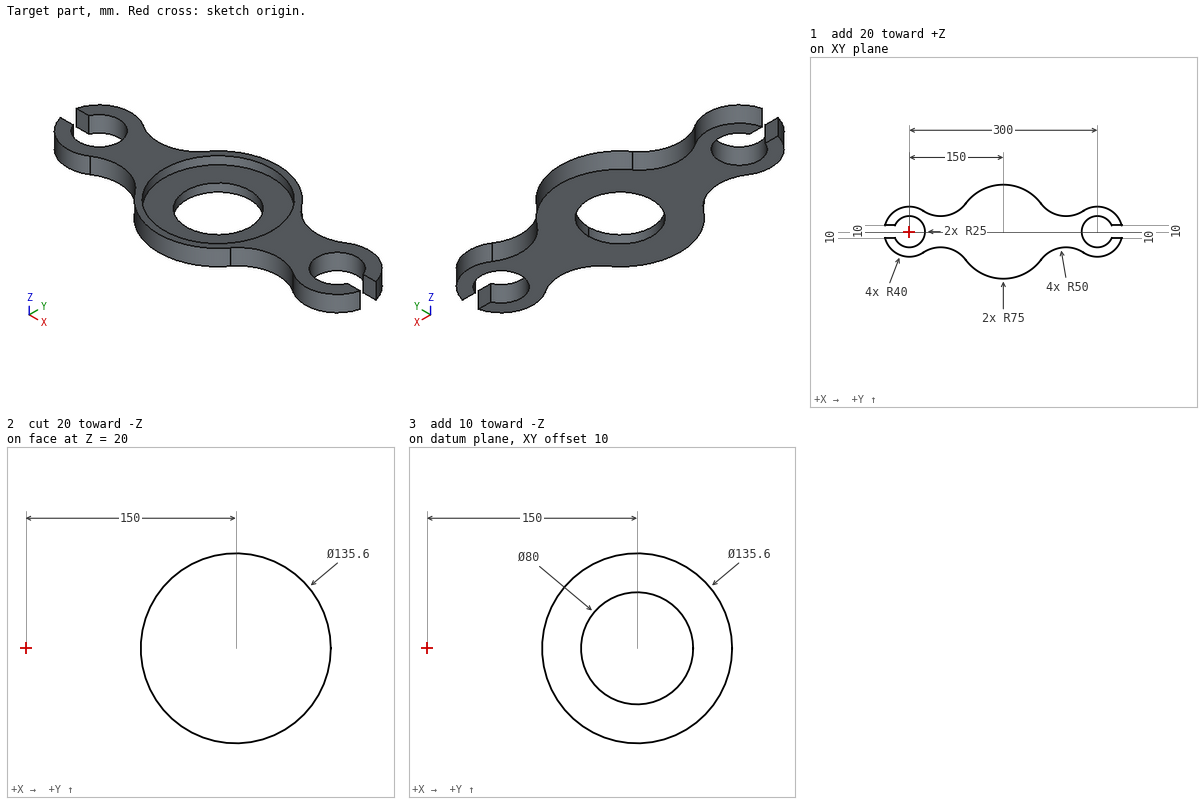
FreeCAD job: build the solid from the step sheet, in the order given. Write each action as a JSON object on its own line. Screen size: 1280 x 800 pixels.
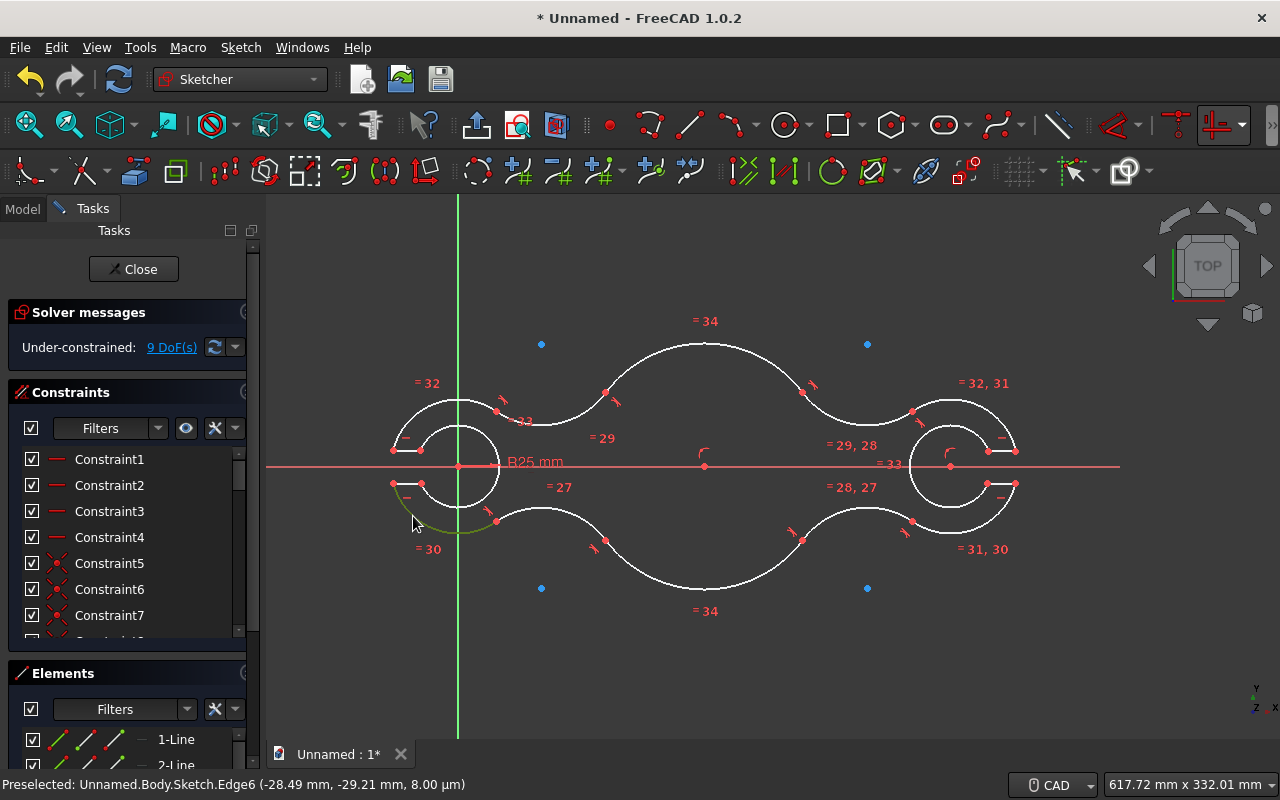
{"action": "key", "text": "k r"}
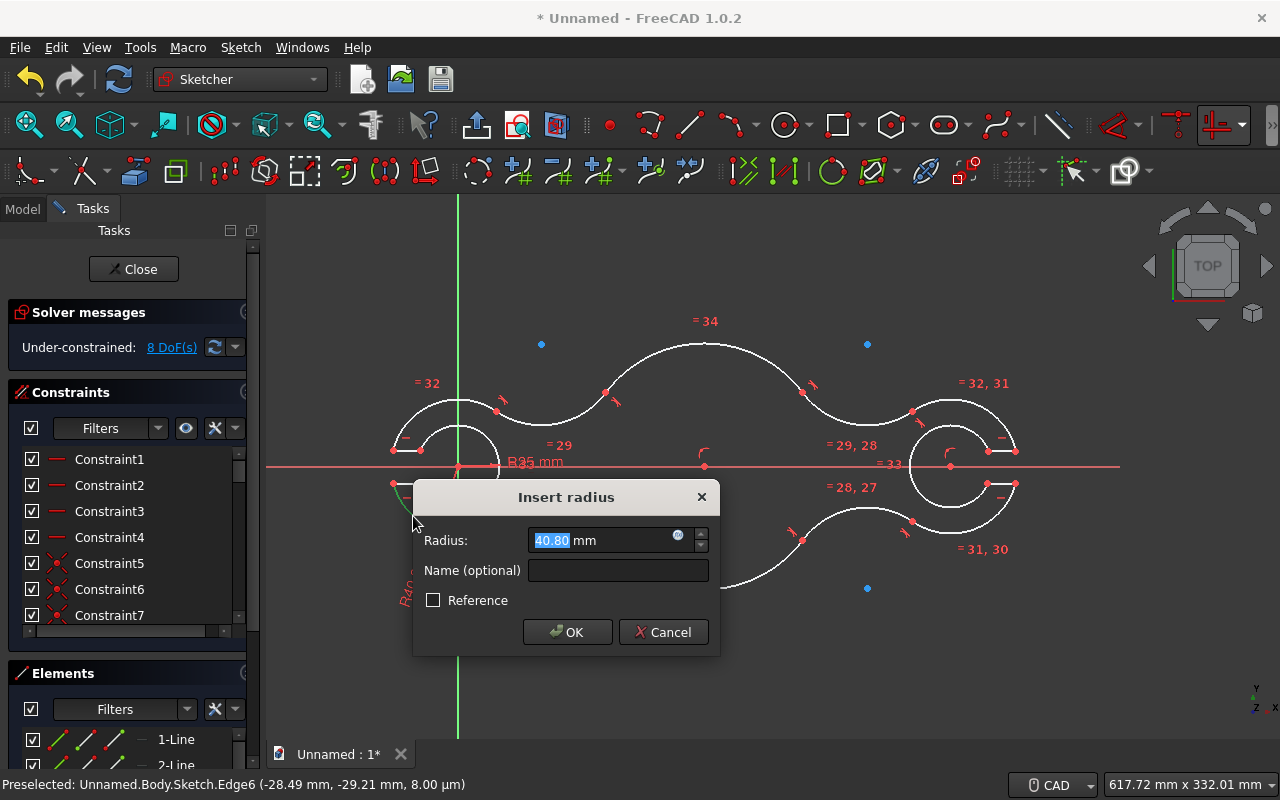
{"action": "type", "text": "40"}
{"action": "key", "text": "Return"}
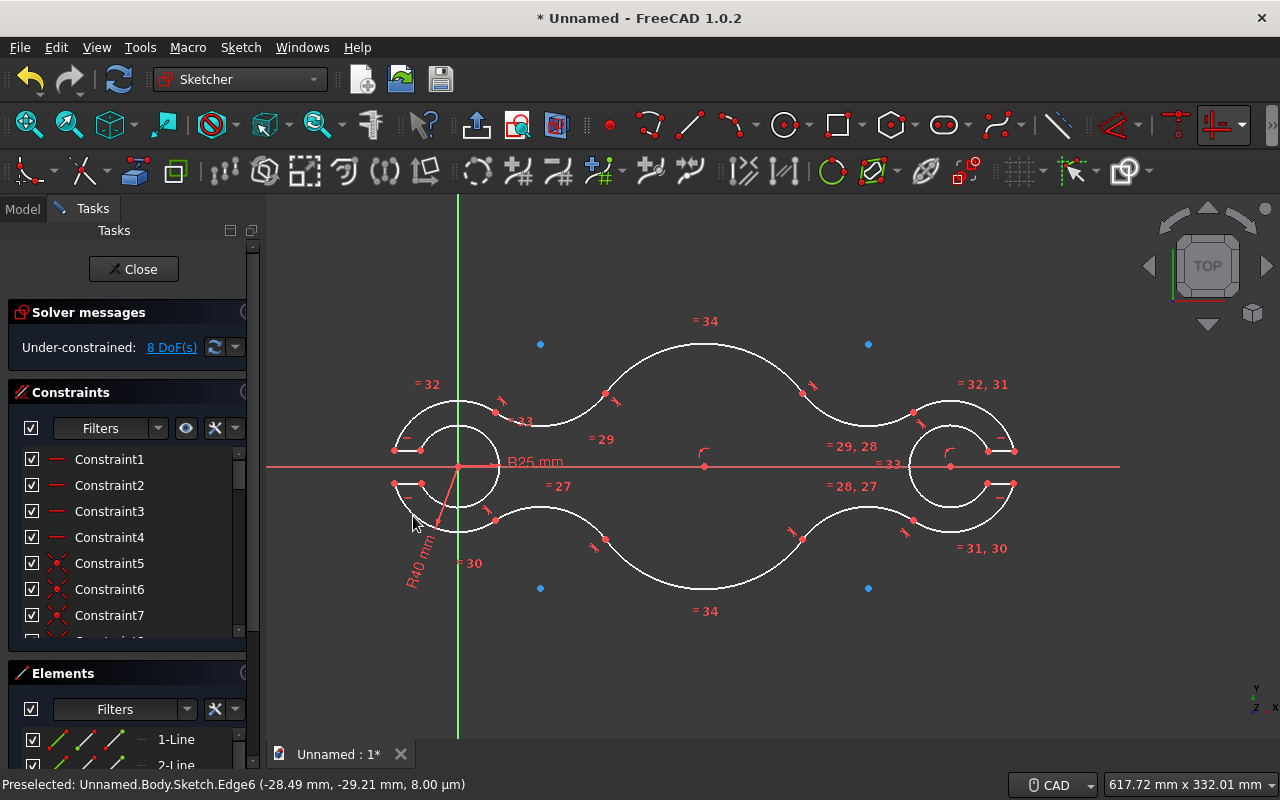
{"action": "left_click", "coordinate": [578, 516]}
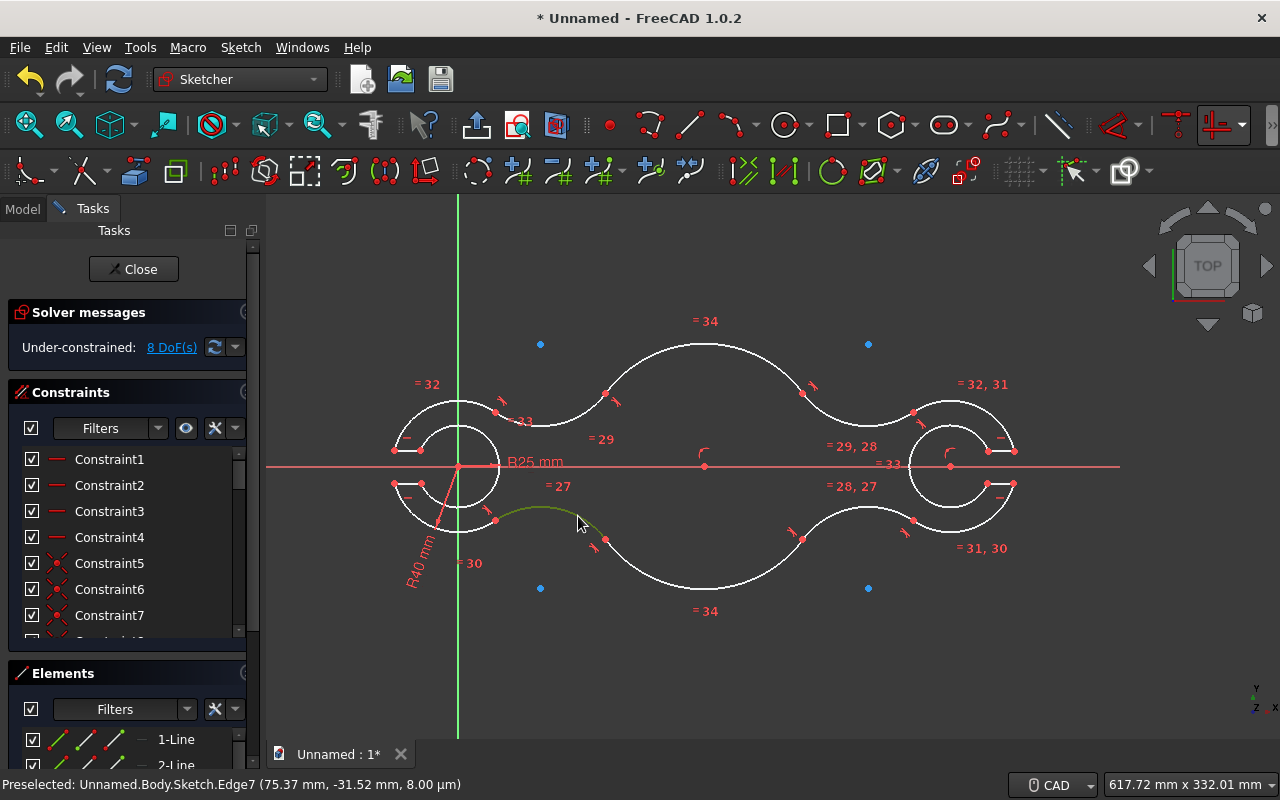
{"action": "left_click", "coordinate": [1140, 126]}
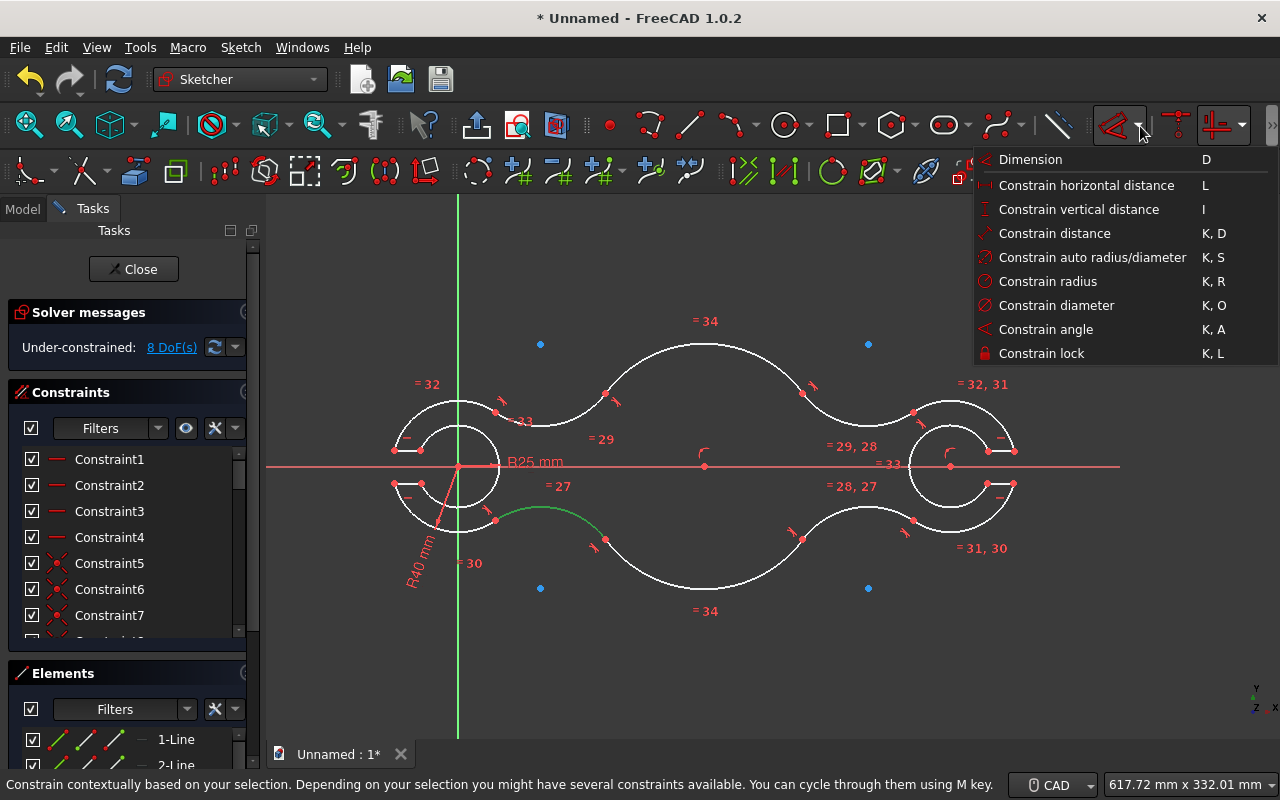
{"action": "left_click", "coordinate": [1126, 281]}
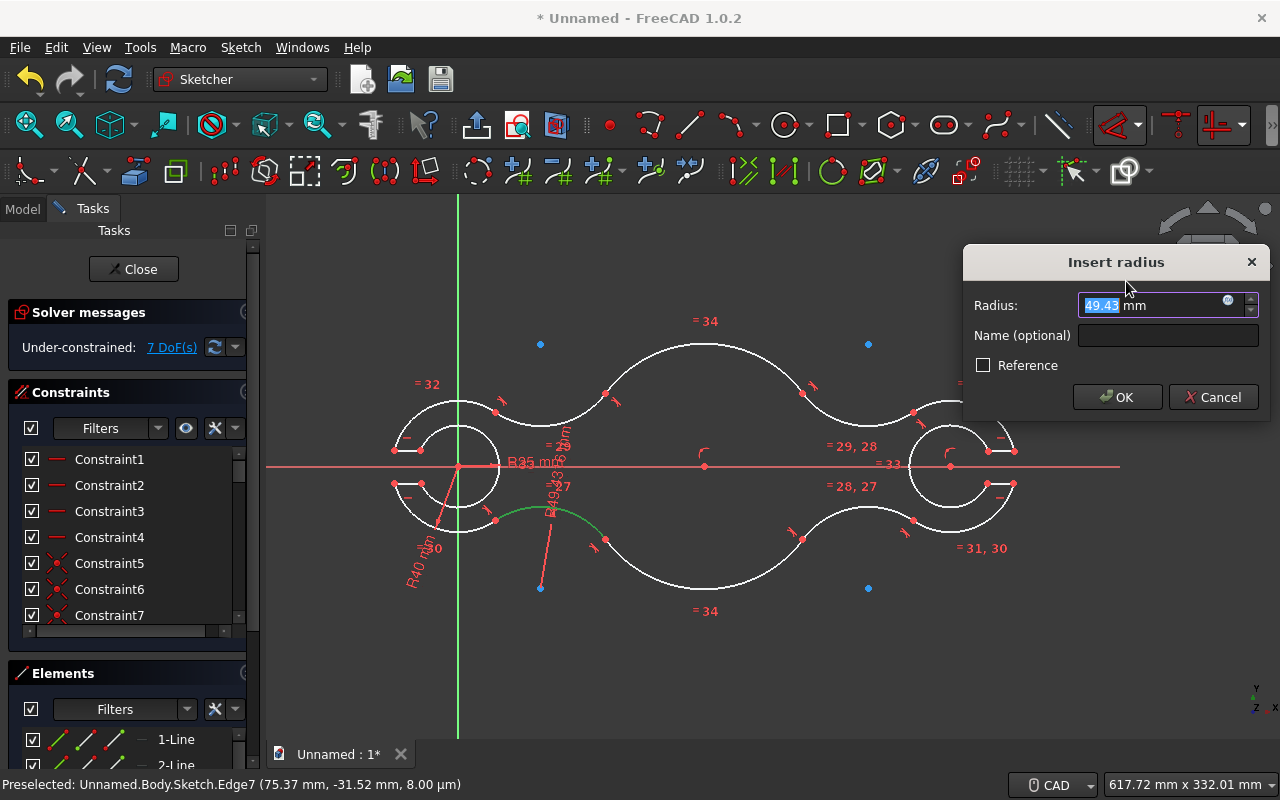
{"action": "type", "text": "50"}
{"action": "key", "text": "Return"}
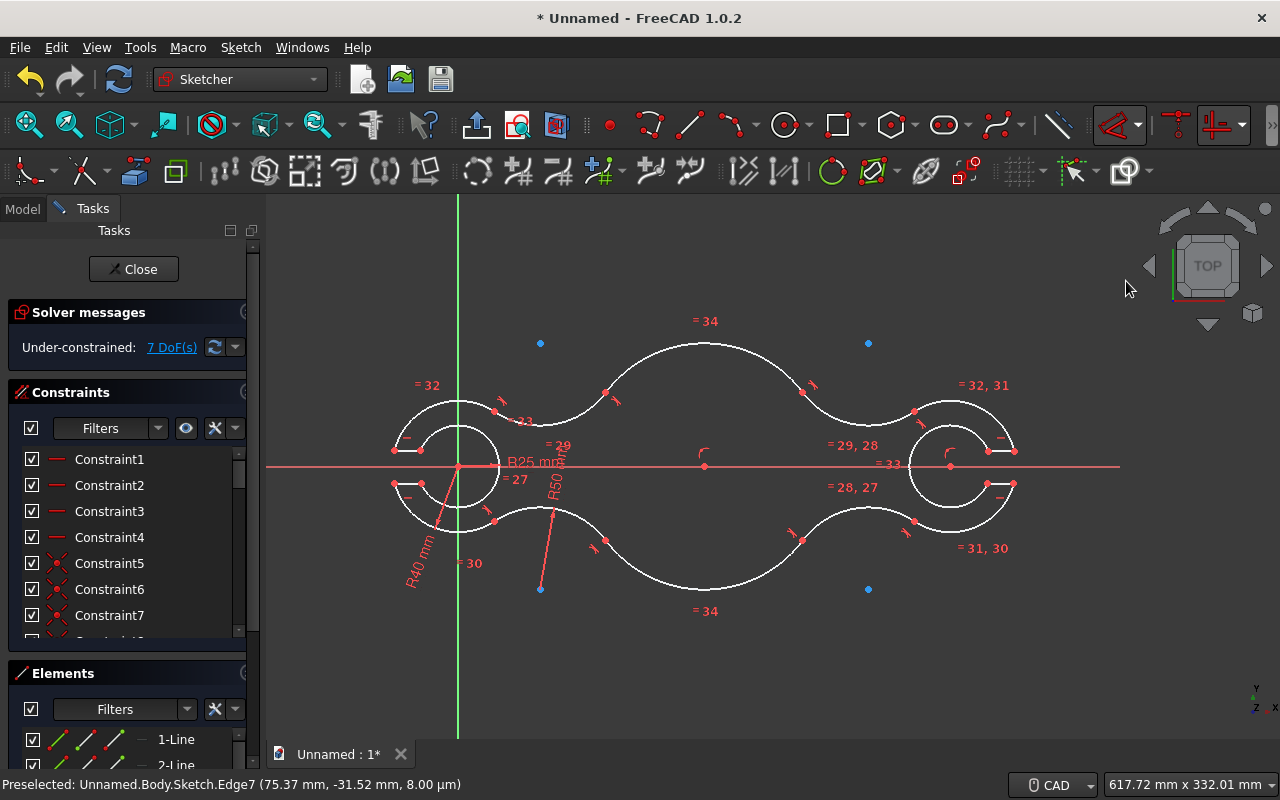
{"action": "left_click", "coordinate": [660, 581]}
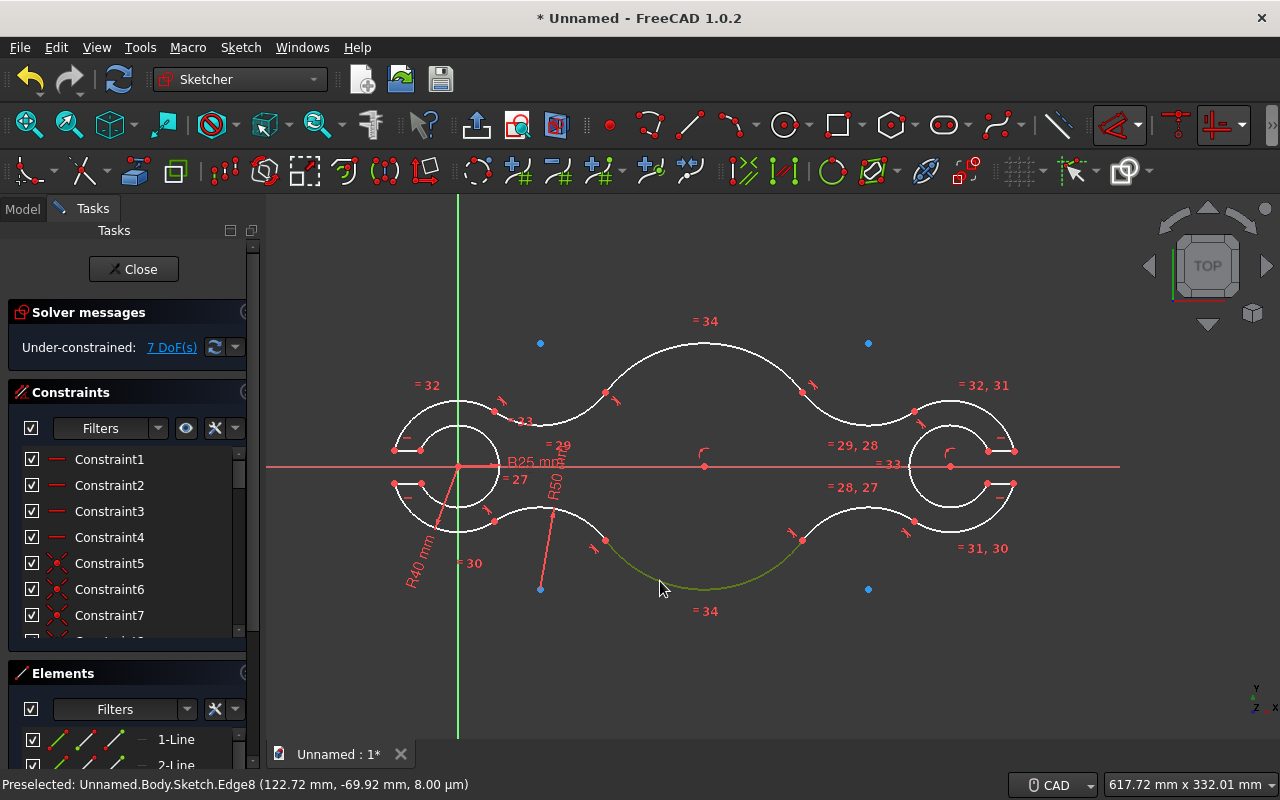
{"action": "left_click", "coordinate": [1140, 126]}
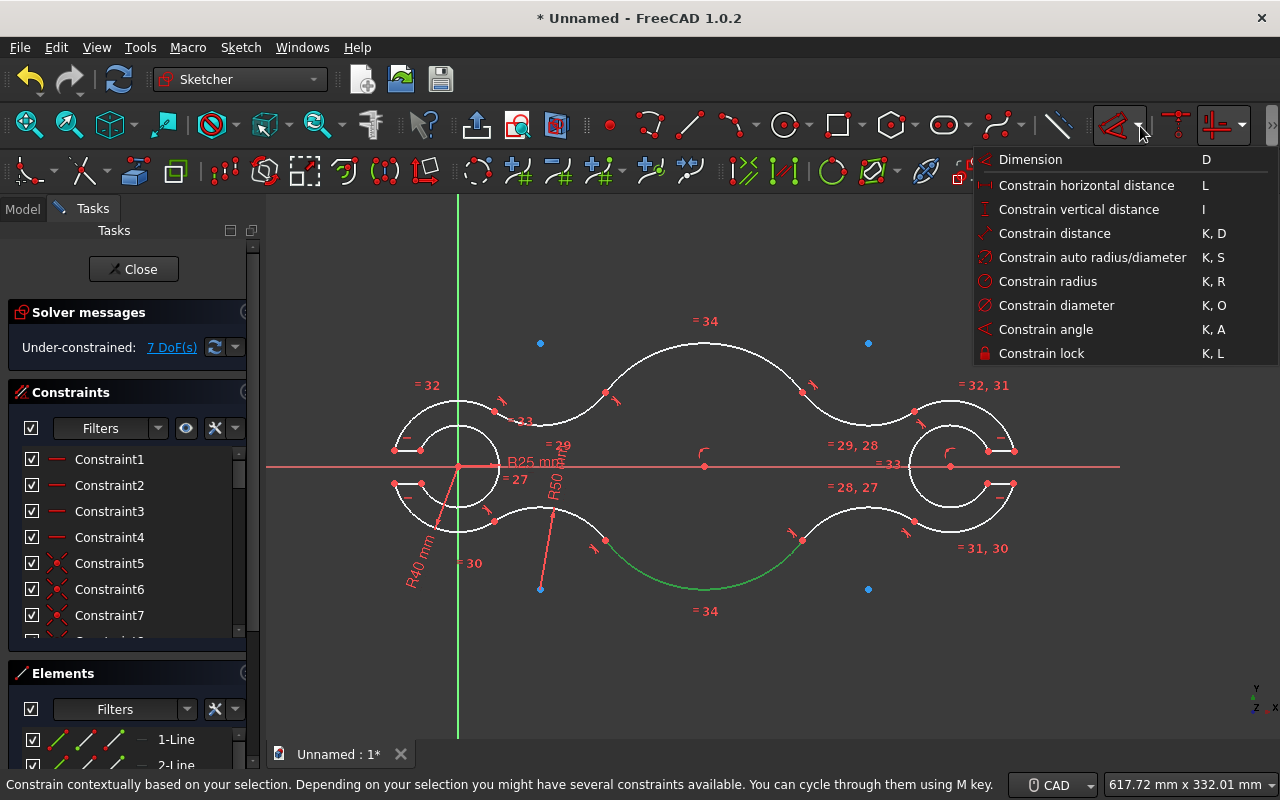
{"action": "left_click", "coordinate": [1126, 281]}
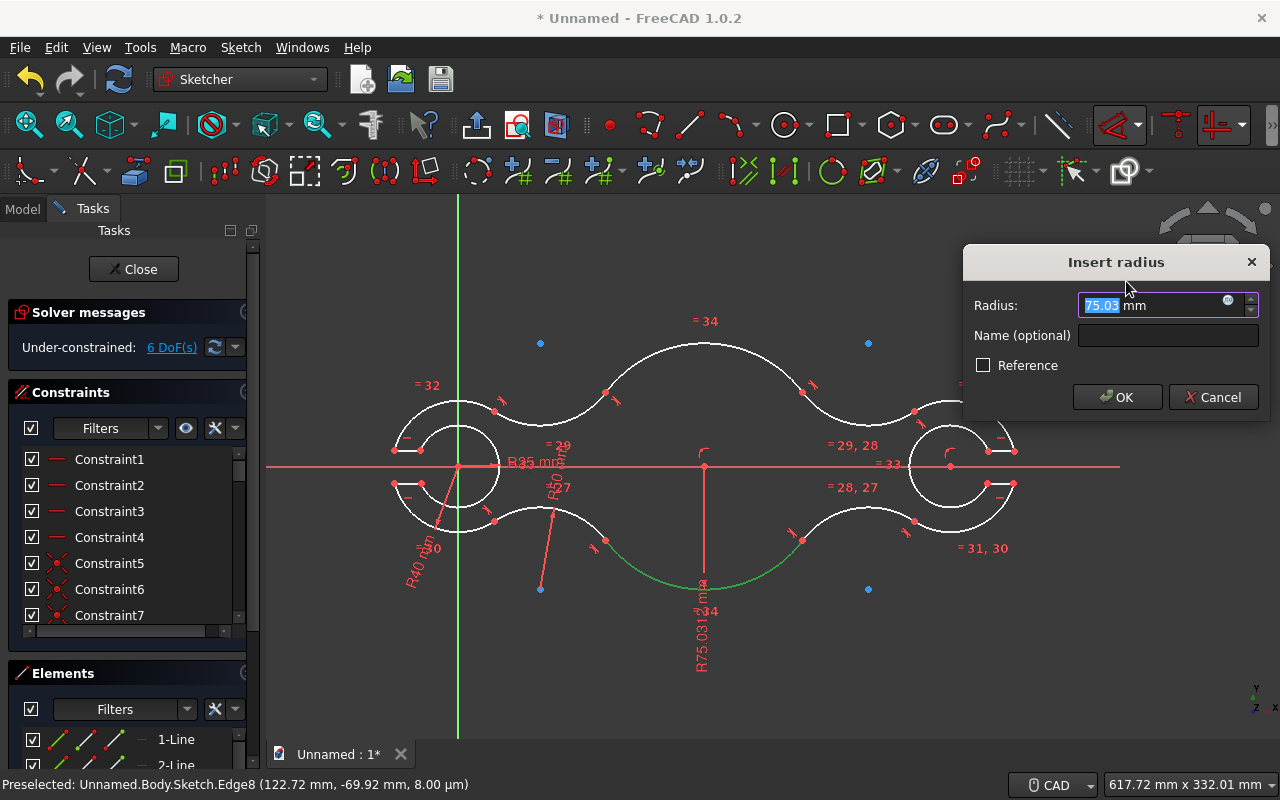
{"action": "type", "text": "75"}
{"action": "key", "text": "Return"}